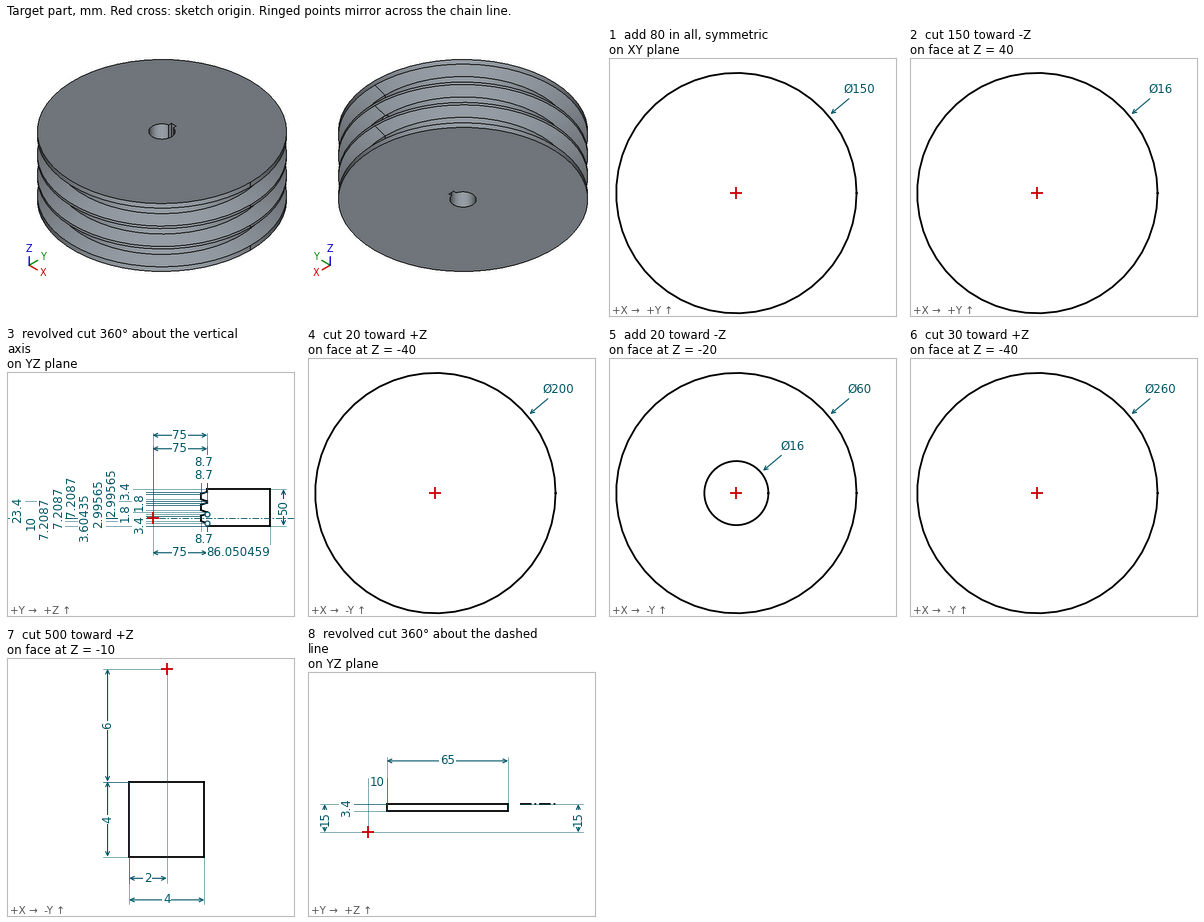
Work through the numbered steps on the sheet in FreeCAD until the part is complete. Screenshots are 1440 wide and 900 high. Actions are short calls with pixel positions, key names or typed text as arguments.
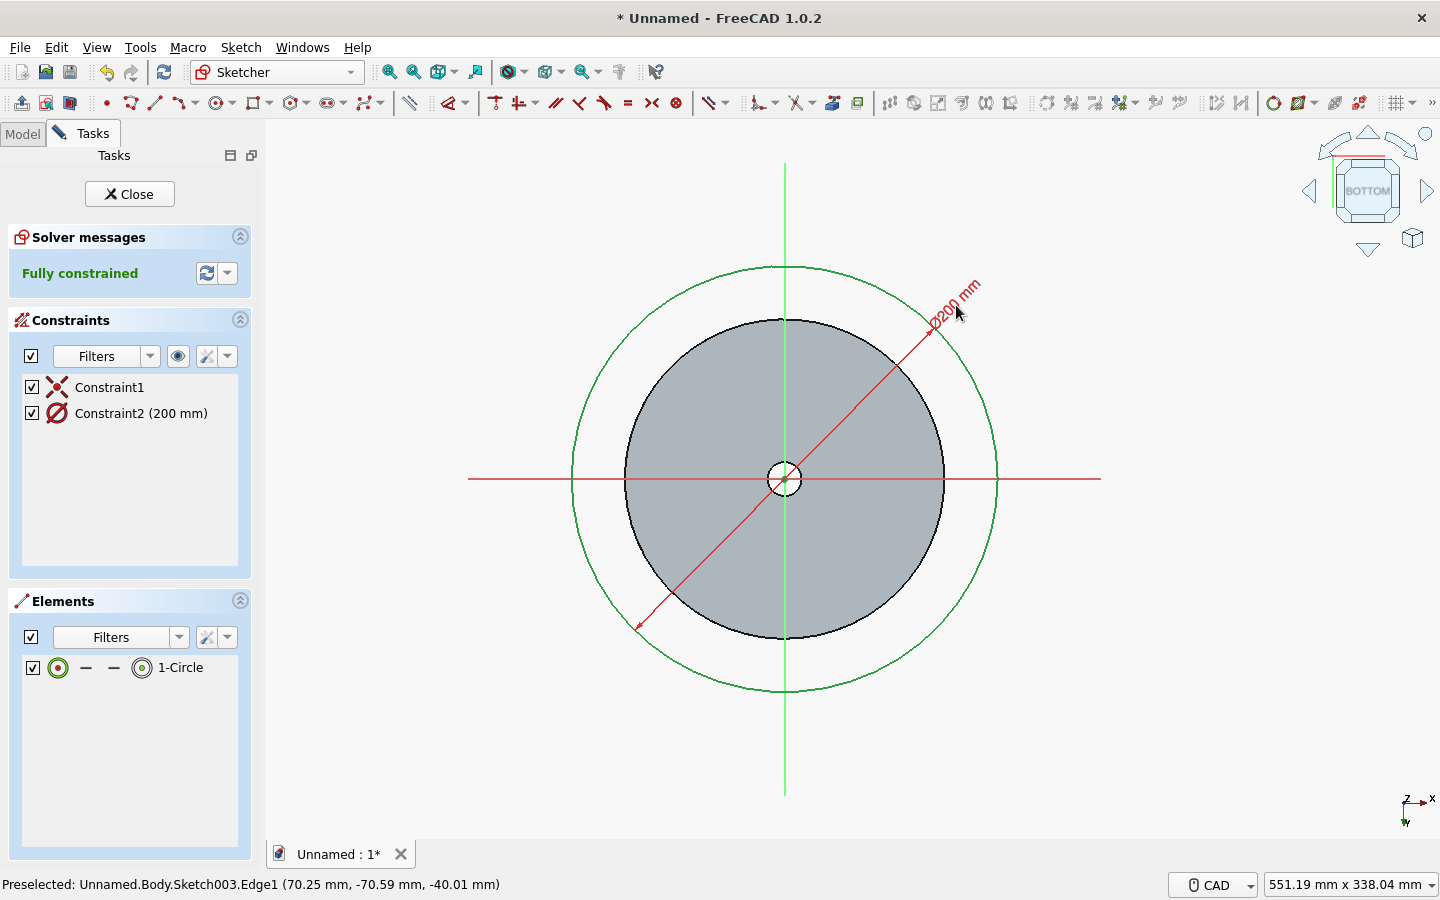
click(130, 194)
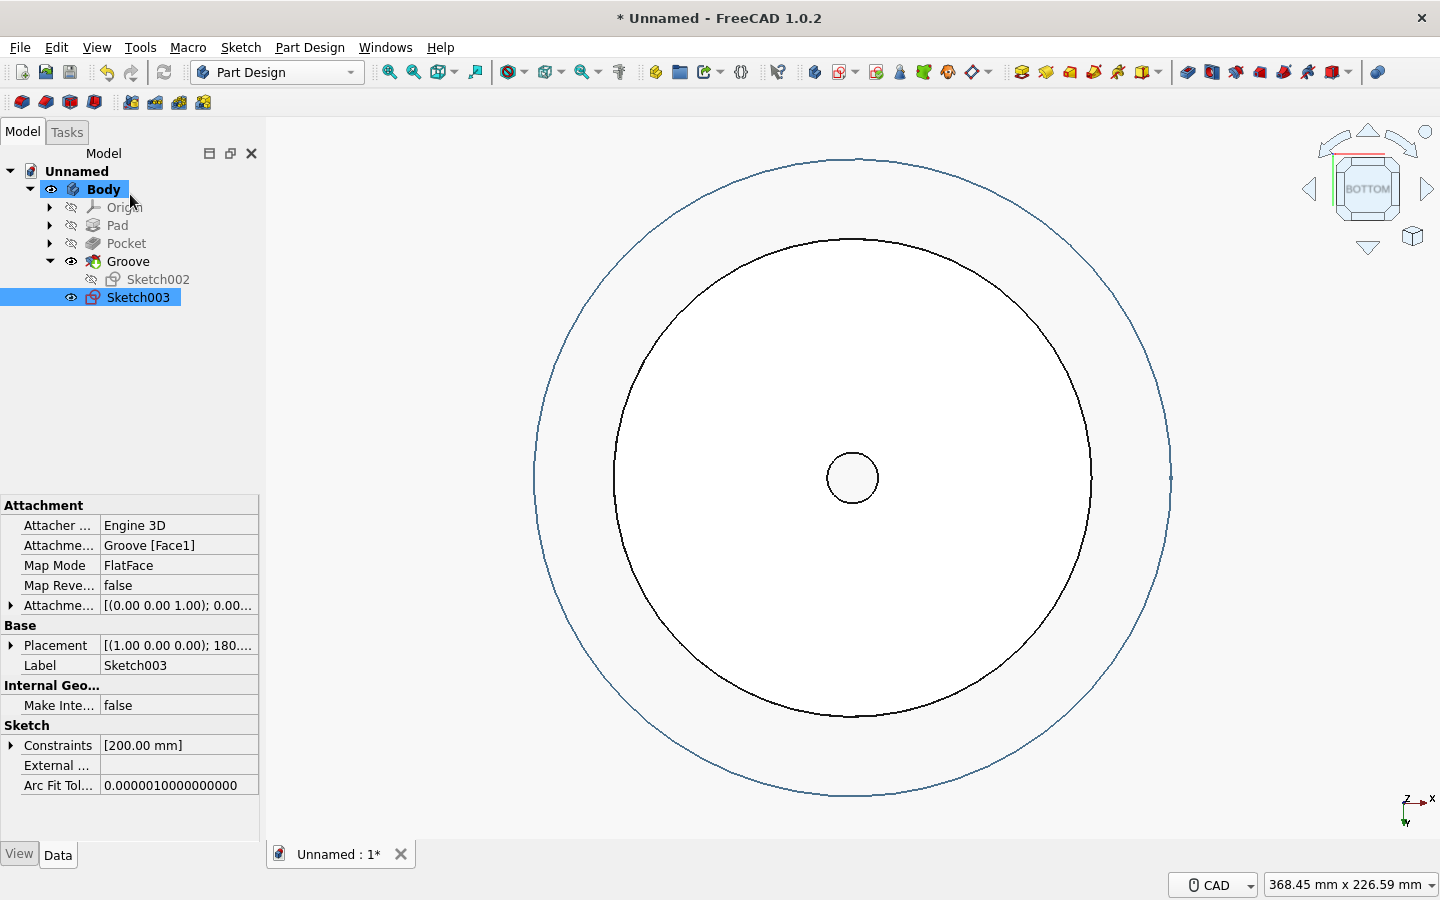
click(1188, 72)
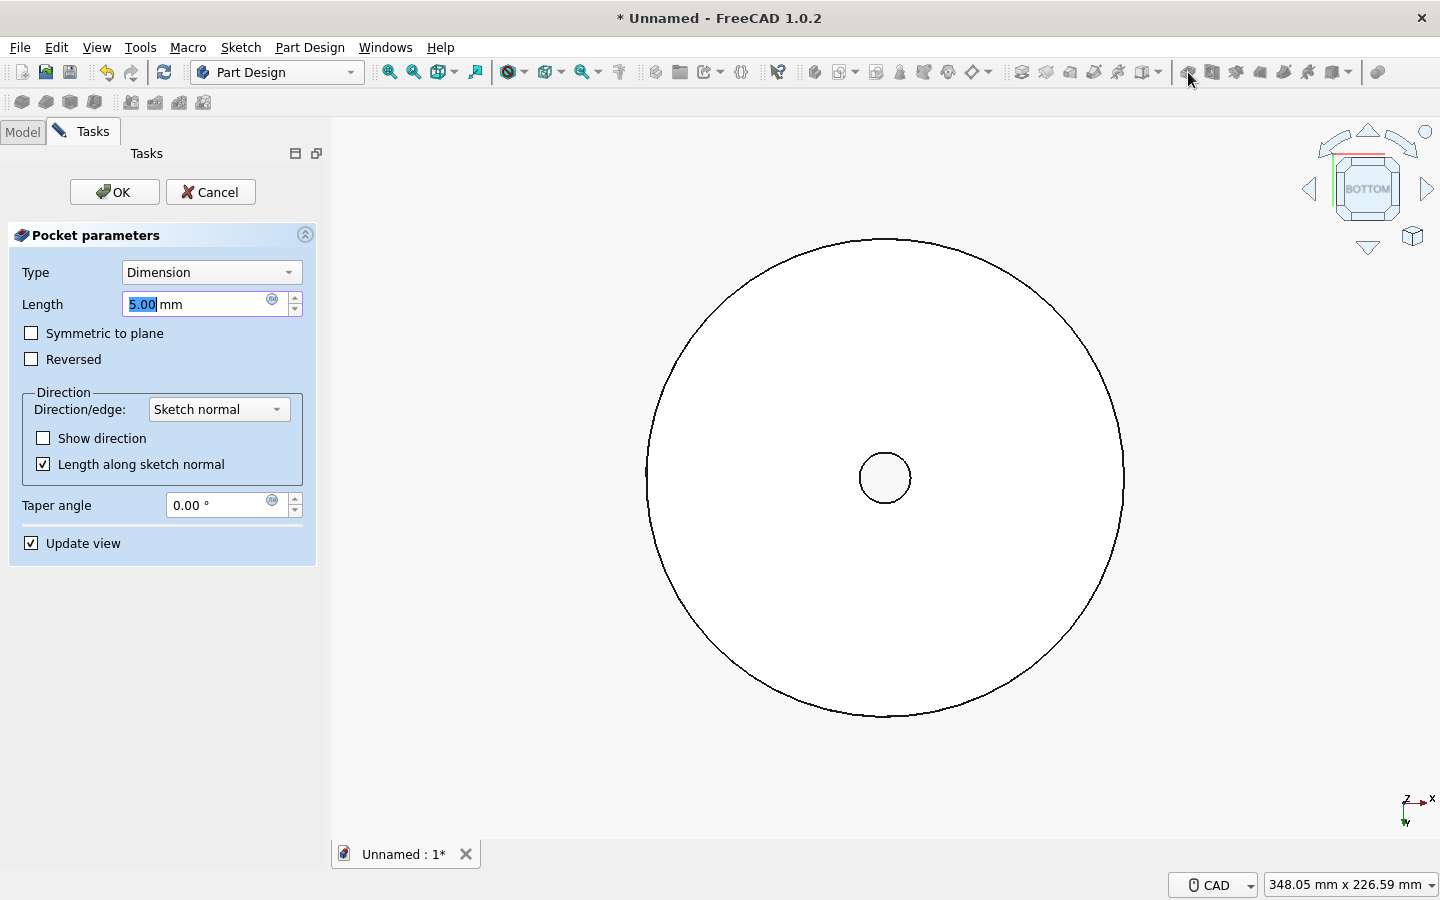
text(20)
key(Tab)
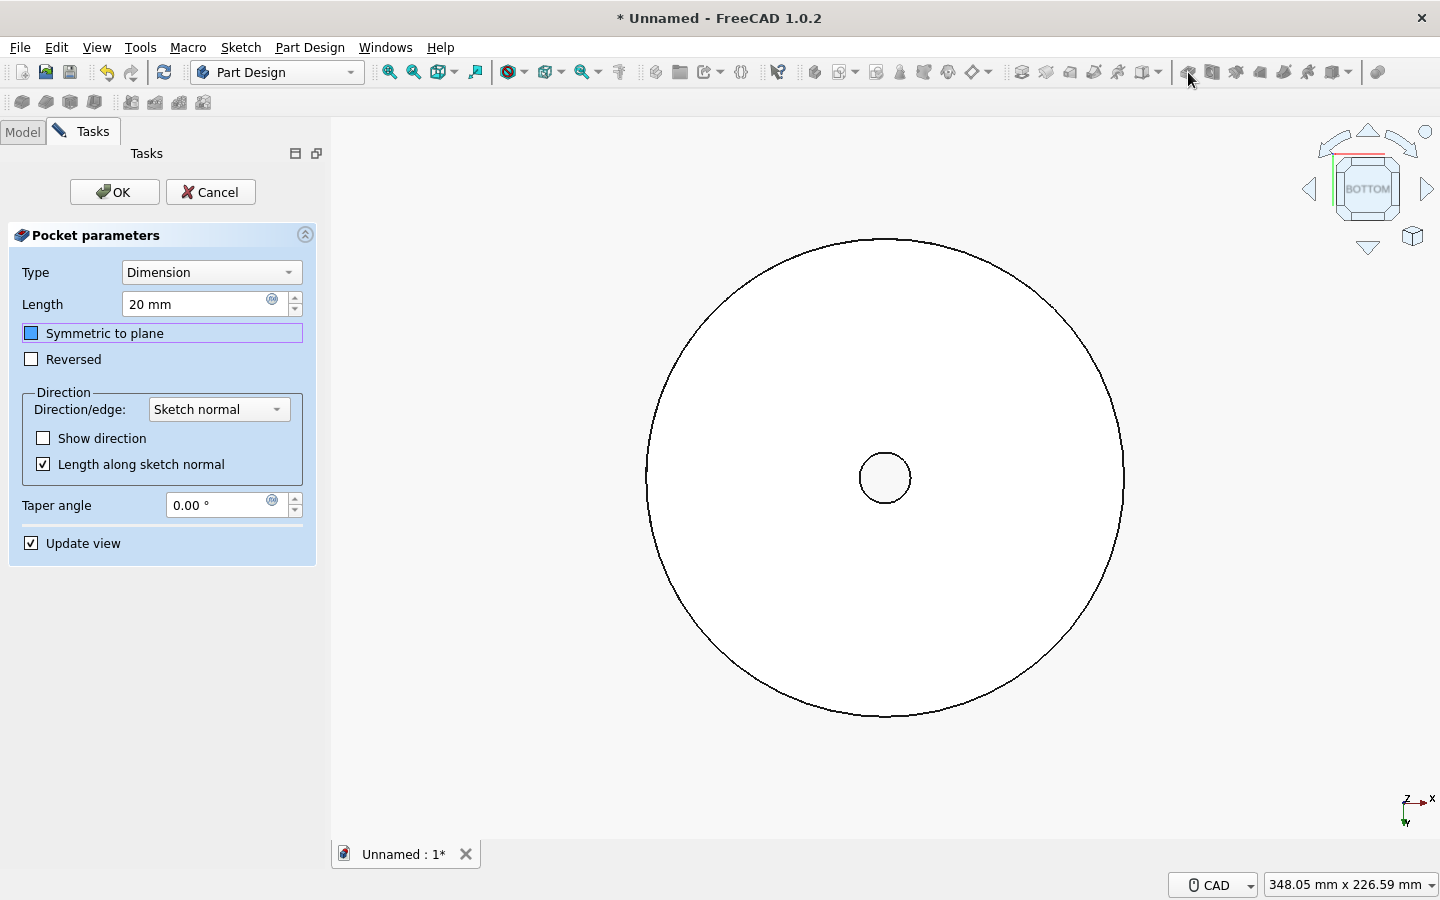
click(115, 192)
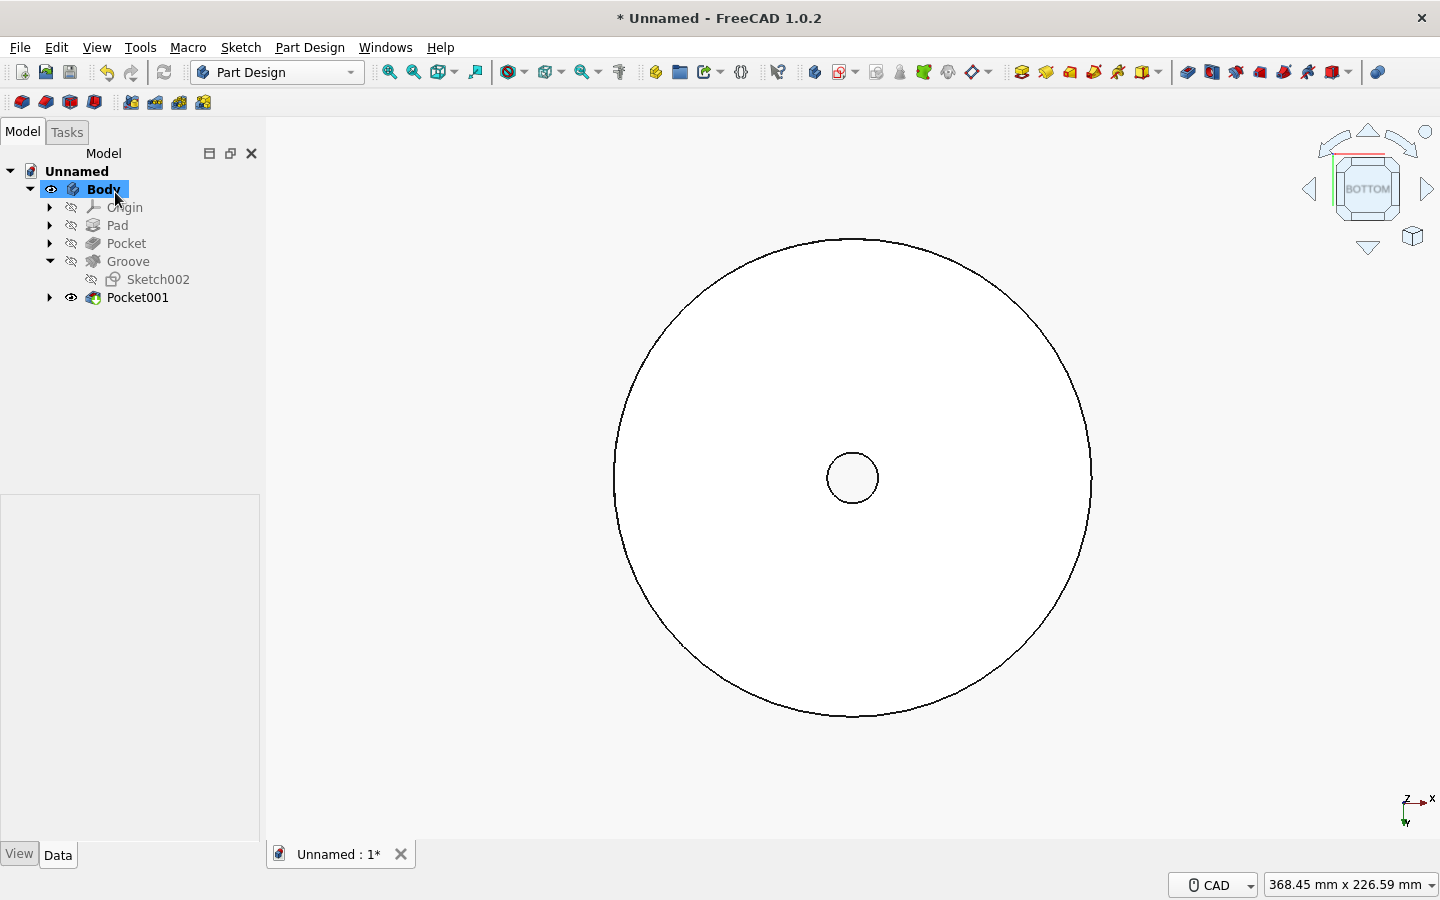
click(853, 613)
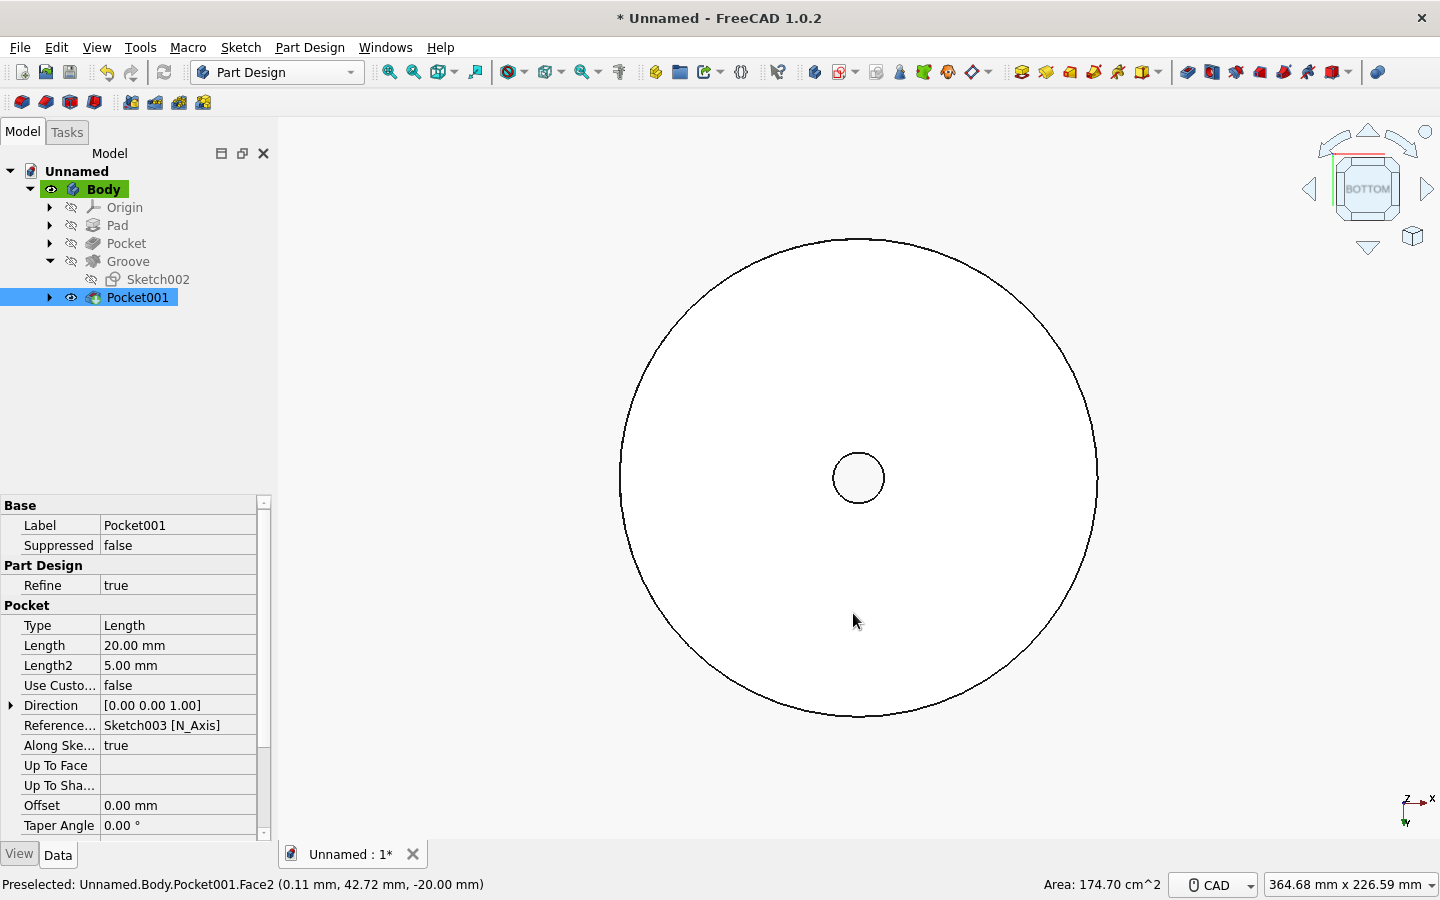
click(840, 72)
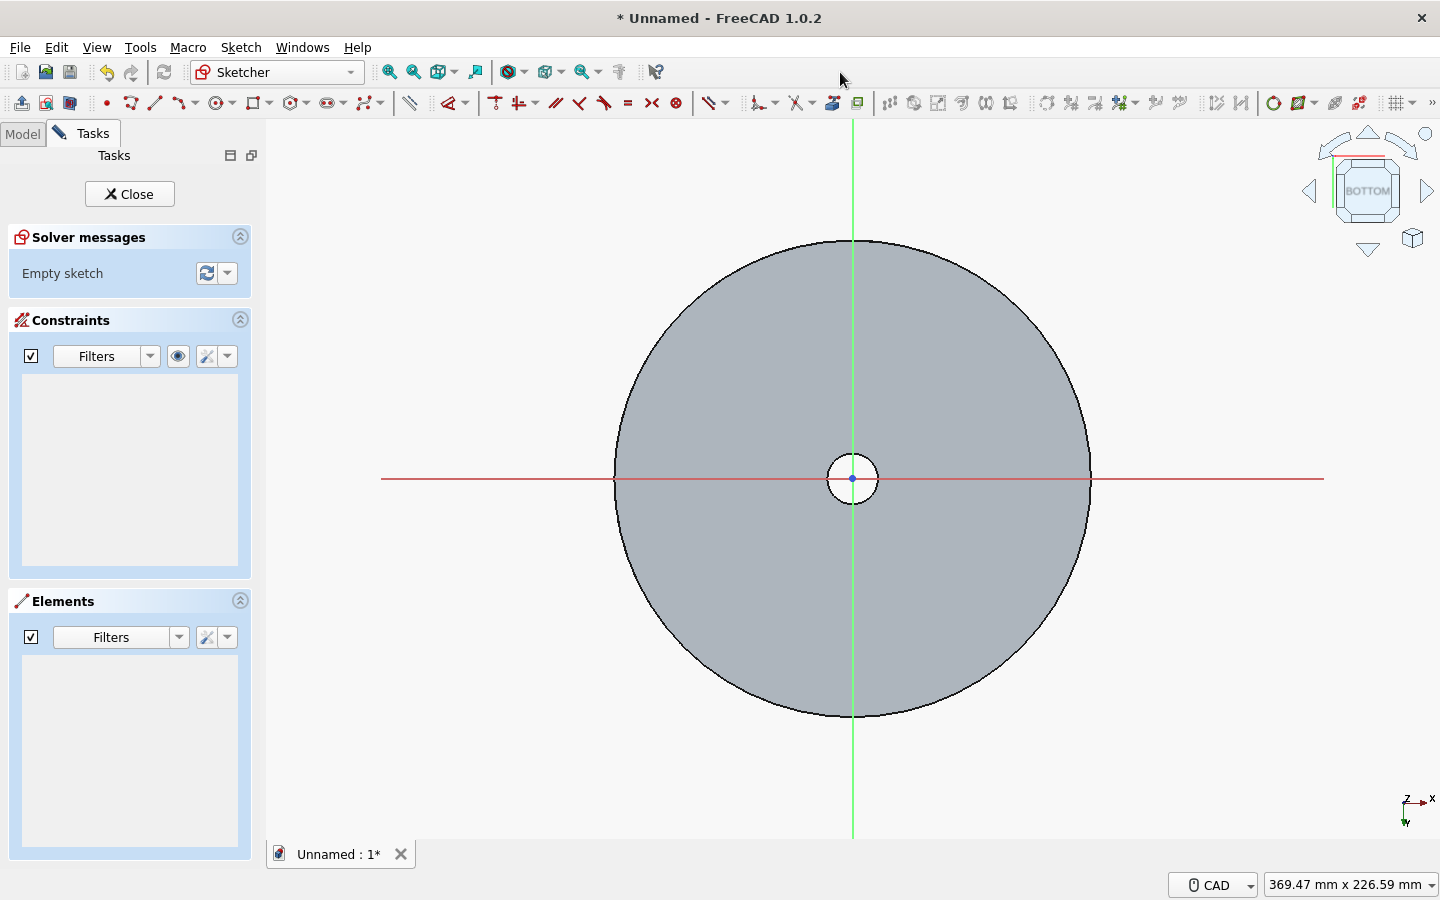
scroll(908, 479, up, 4)